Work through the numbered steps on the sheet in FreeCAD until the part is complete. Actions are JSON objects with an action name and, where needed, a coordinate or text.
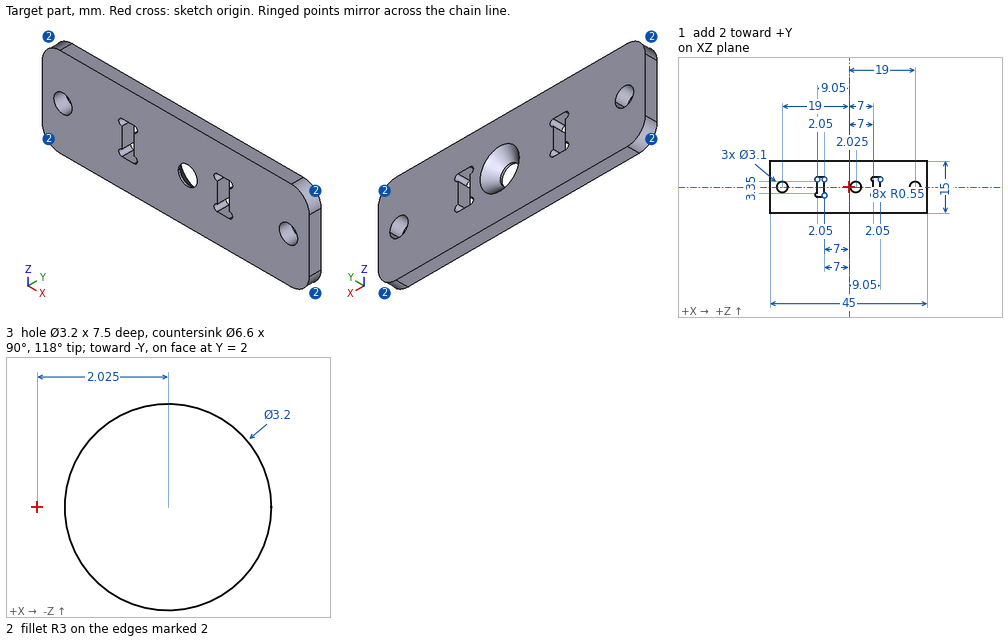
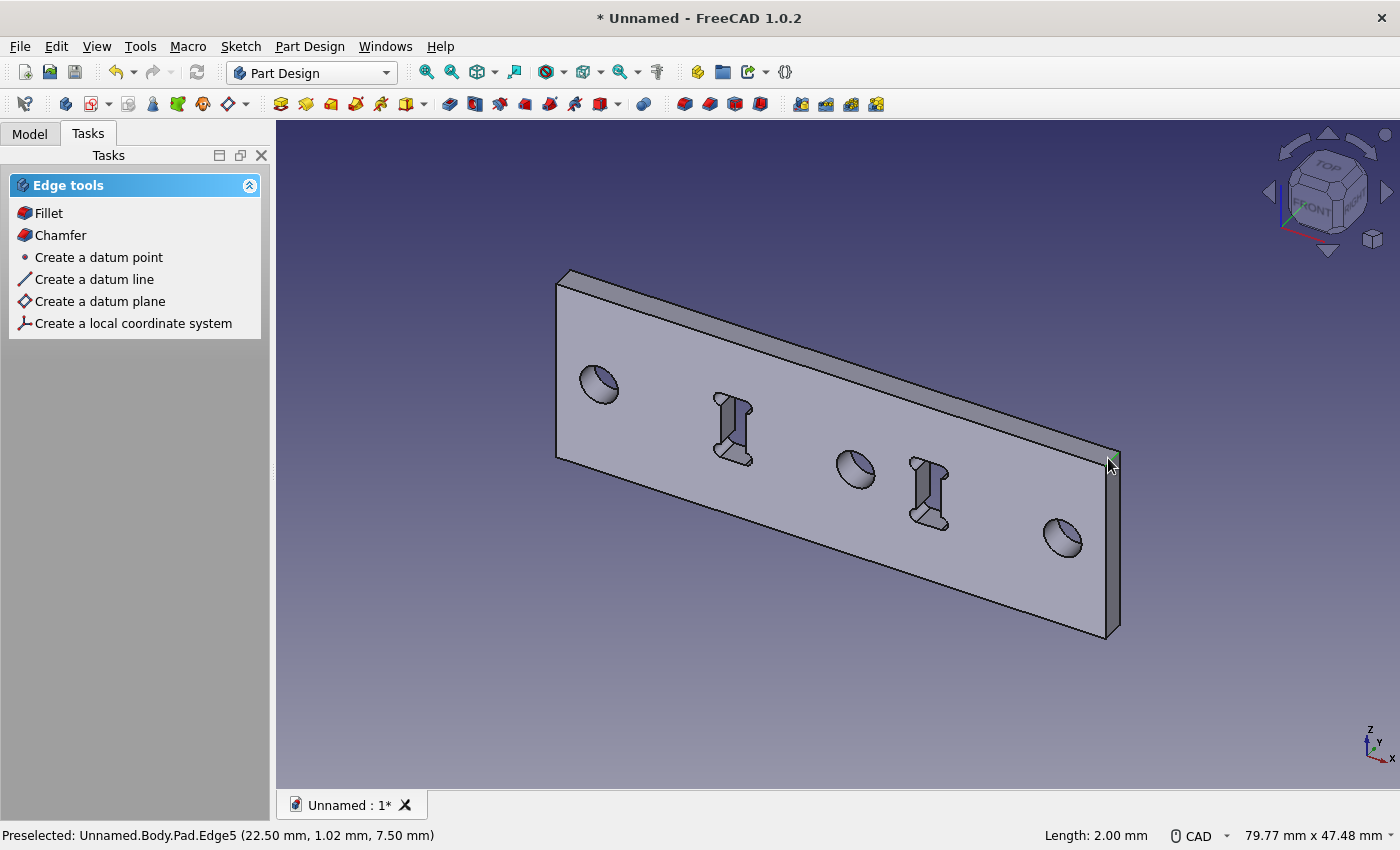
{"action": "key", "text": "0"}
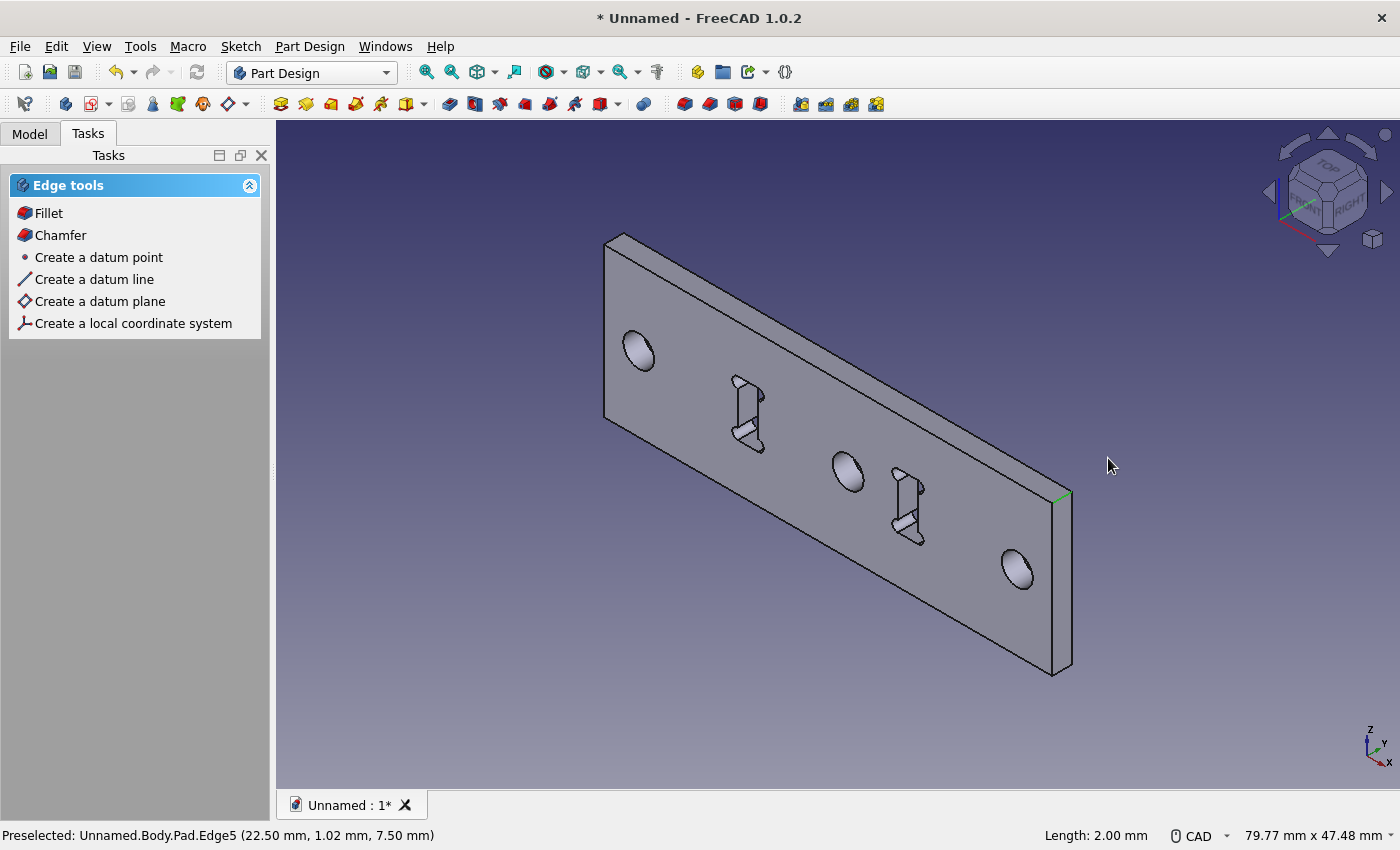
{"action": "key", "text": "2"}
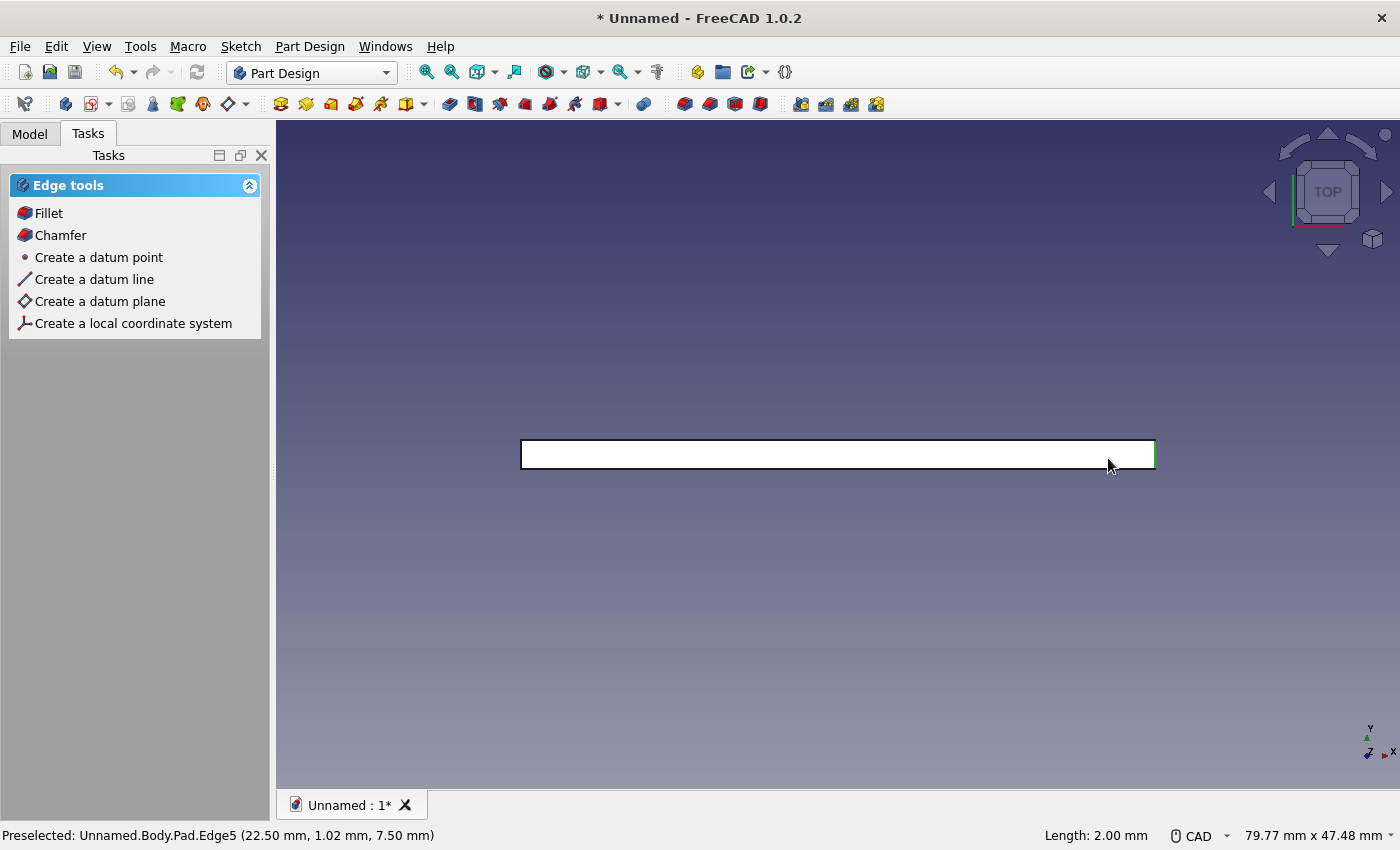
{"action": "left_click", "coordinate": [521, 454], "text": "ctrl"}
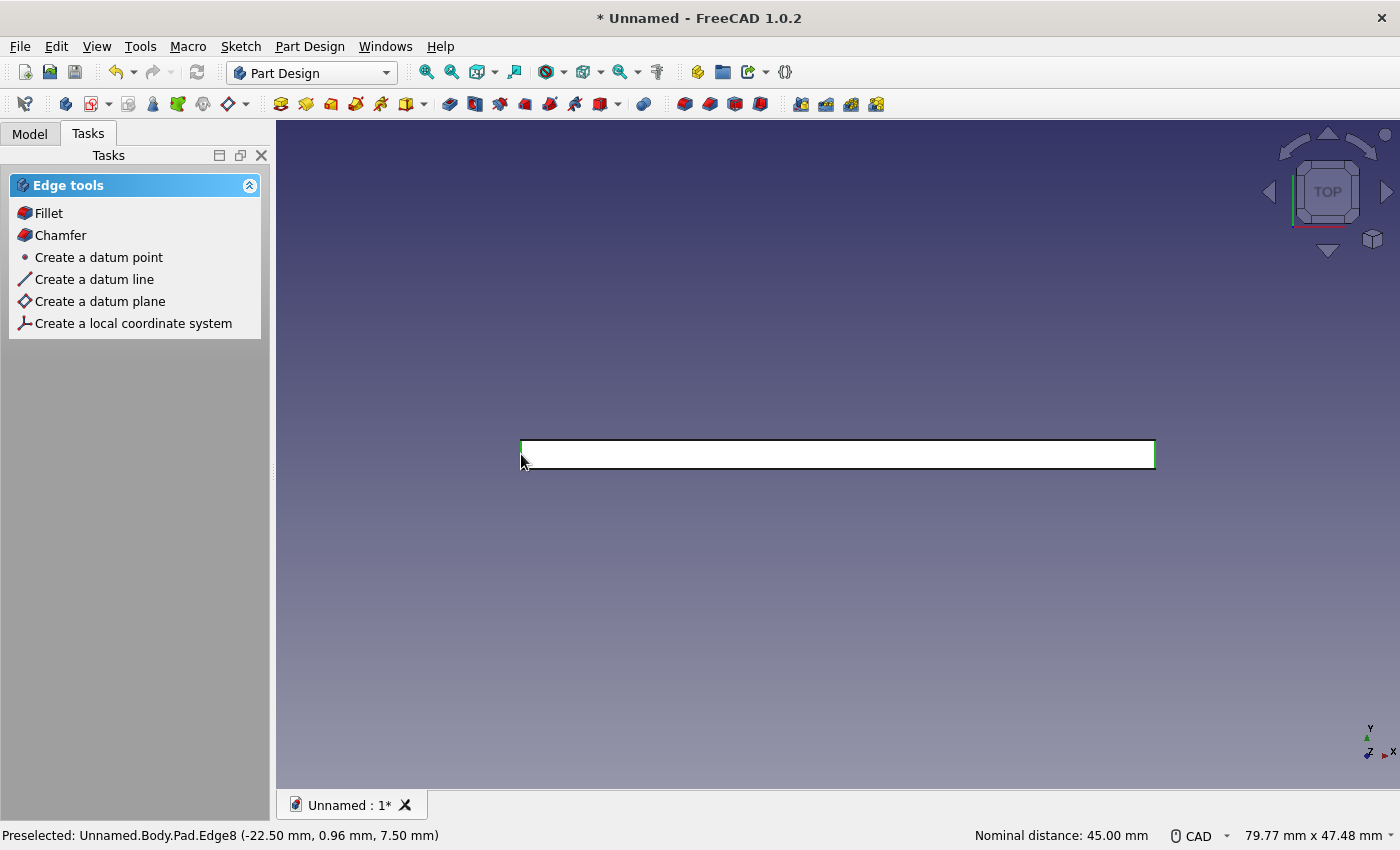
{"action": "key", "text": "1"}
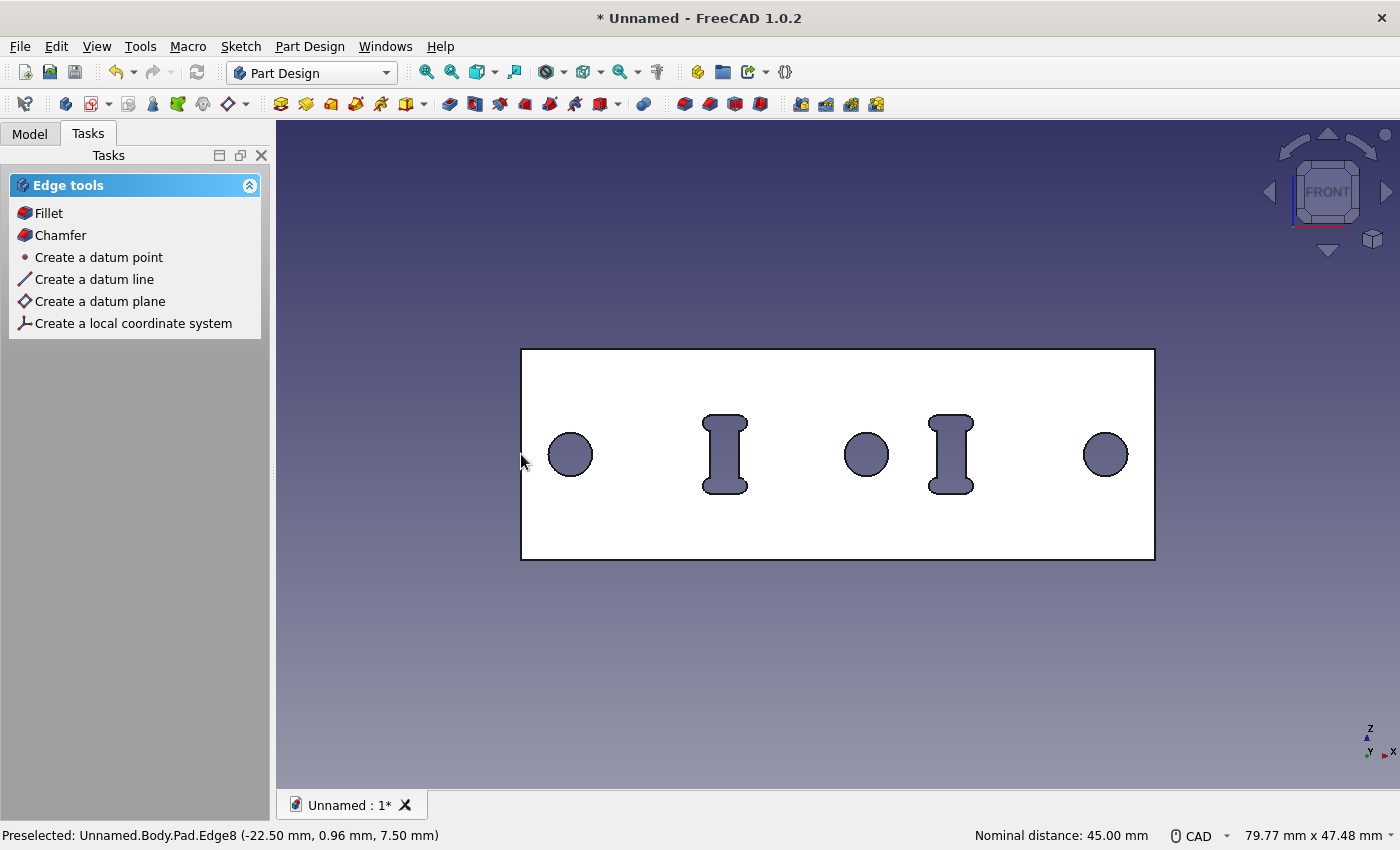
{"action": "key", "text": "3"}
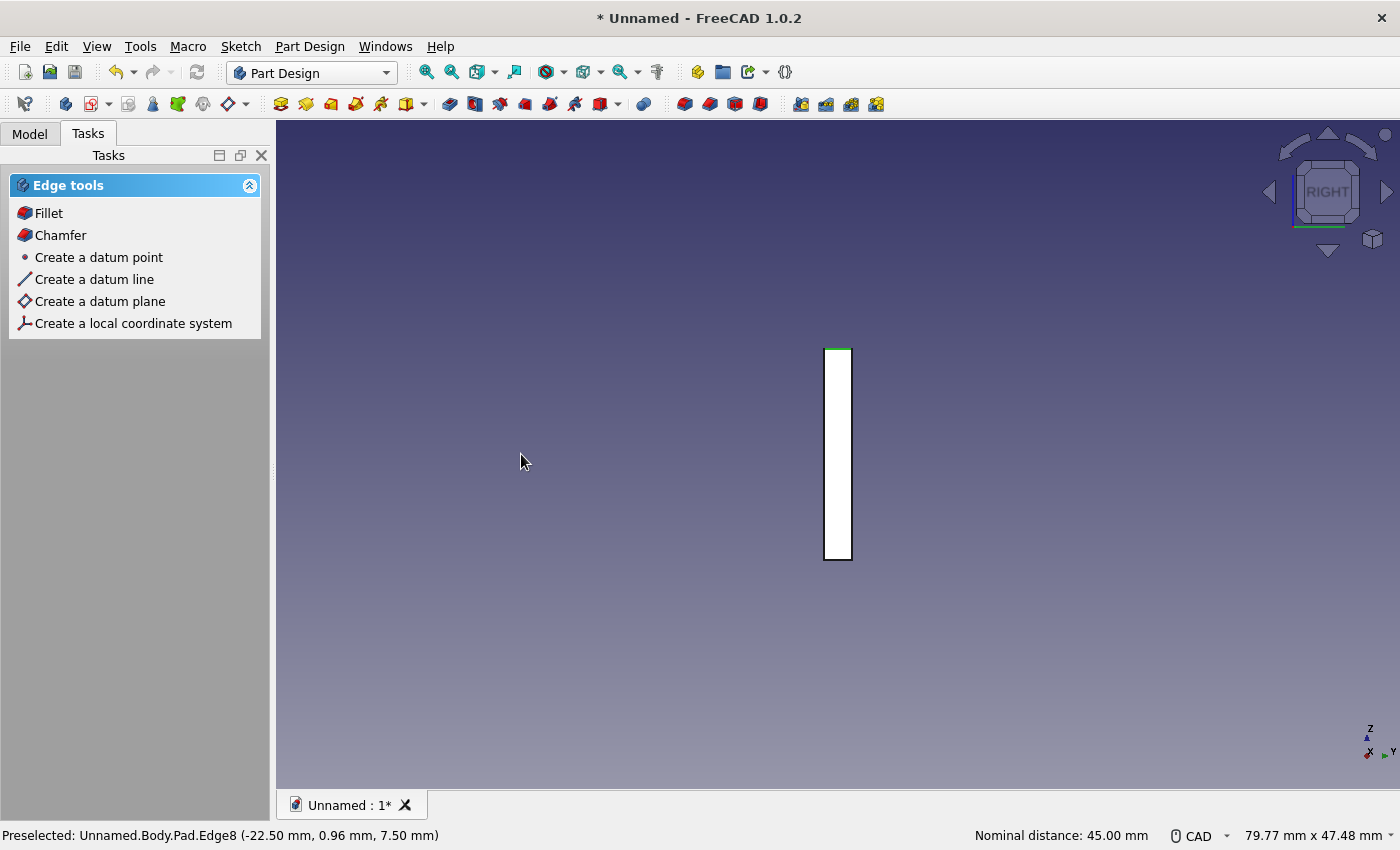
{"action": "left_click", "coordinate": [427, 72]}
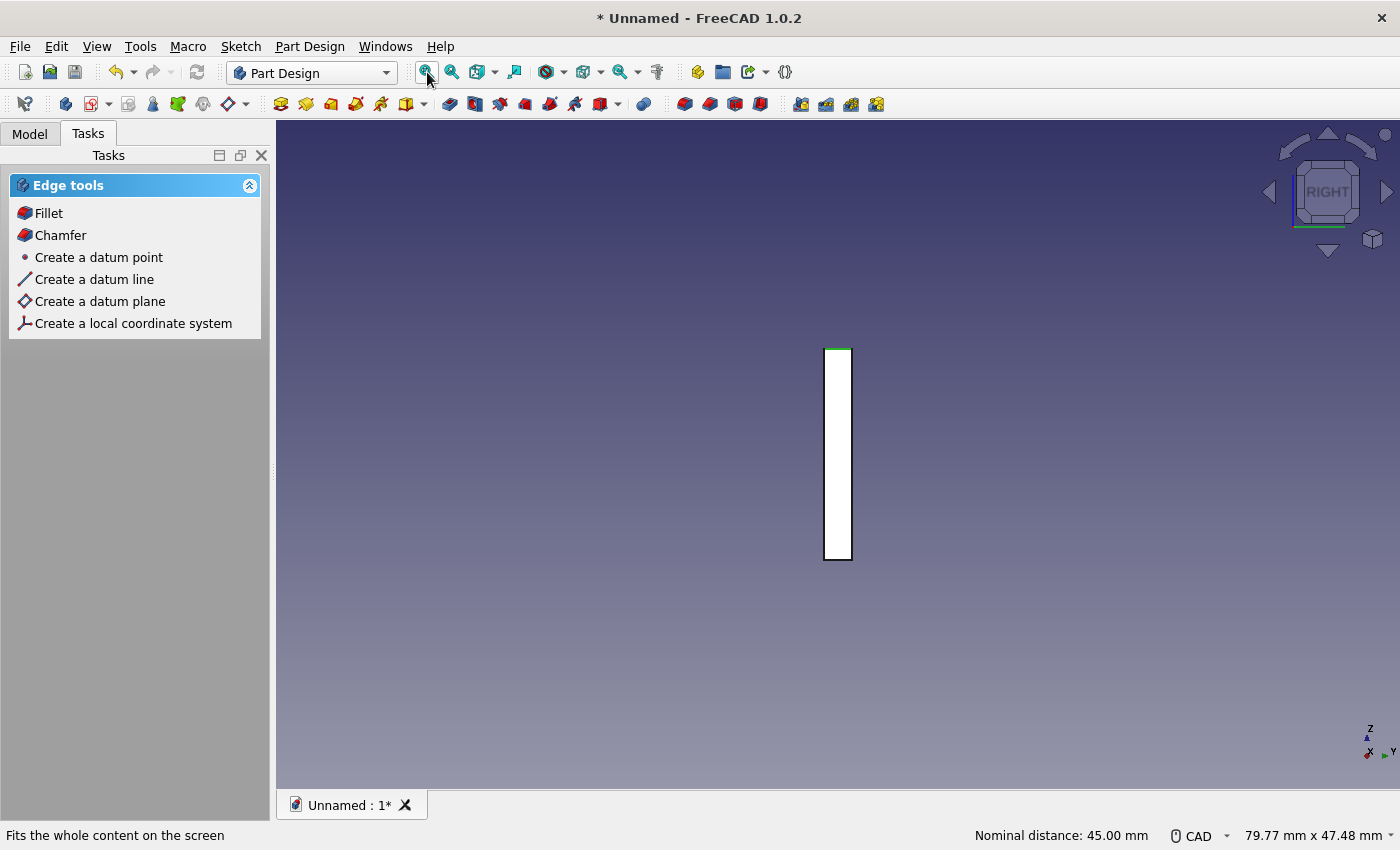
{"action": "left_click", "coordinate": [838, 559], "text": "ctrl"}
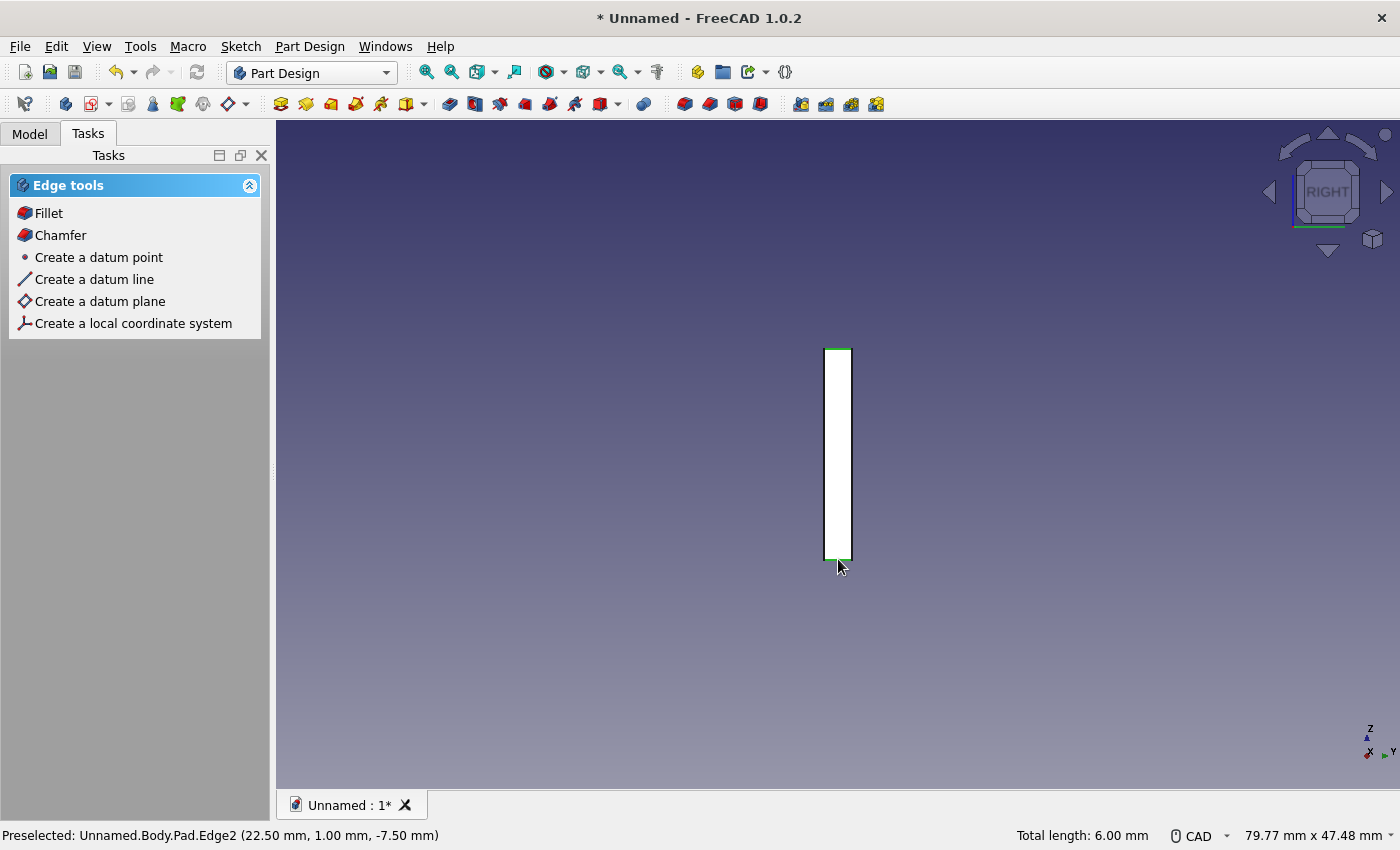
{"action": "key", "text": "5"}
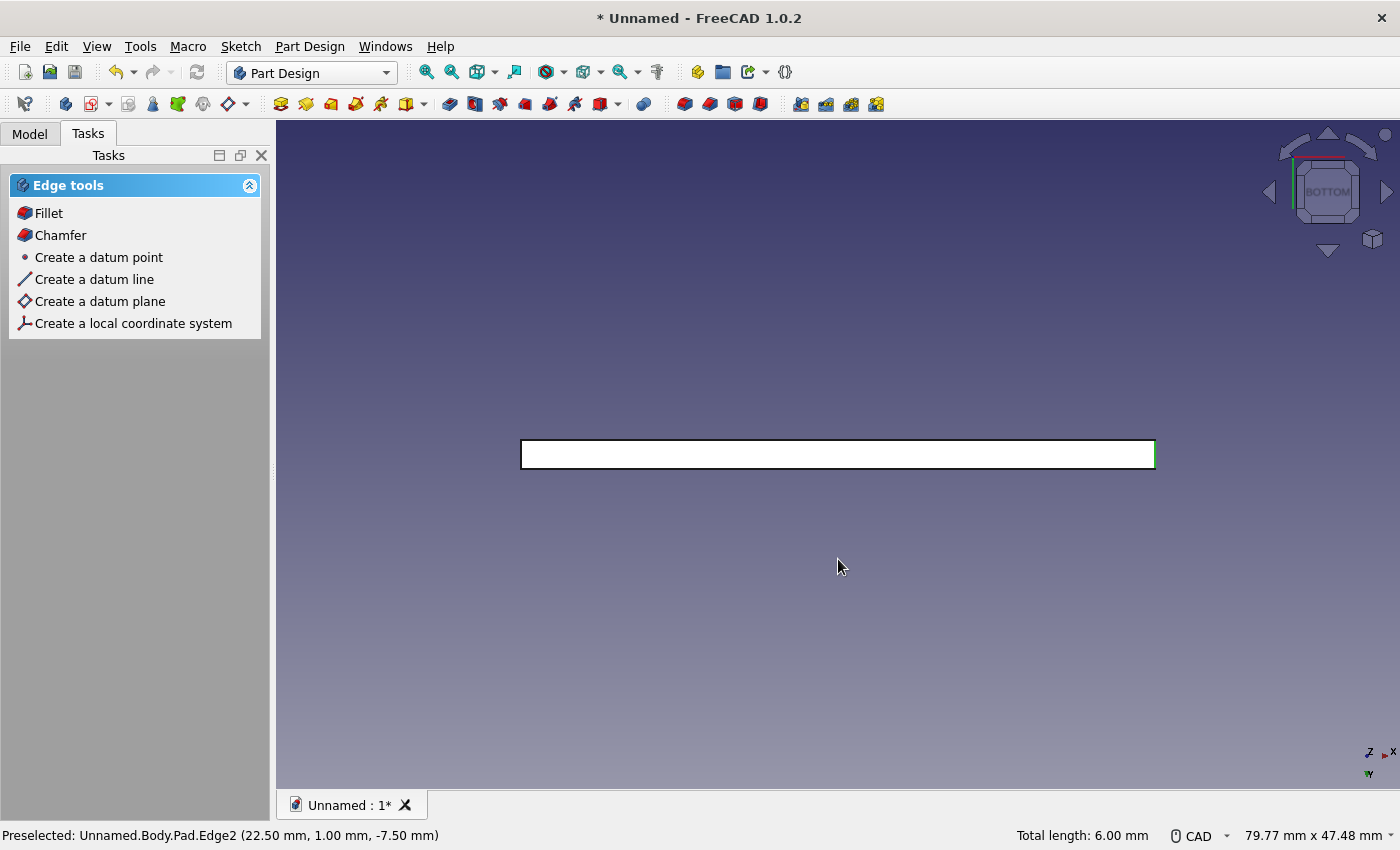
{"action": "left_click", "coordinate": [521, 453], "text": "ctrl"}